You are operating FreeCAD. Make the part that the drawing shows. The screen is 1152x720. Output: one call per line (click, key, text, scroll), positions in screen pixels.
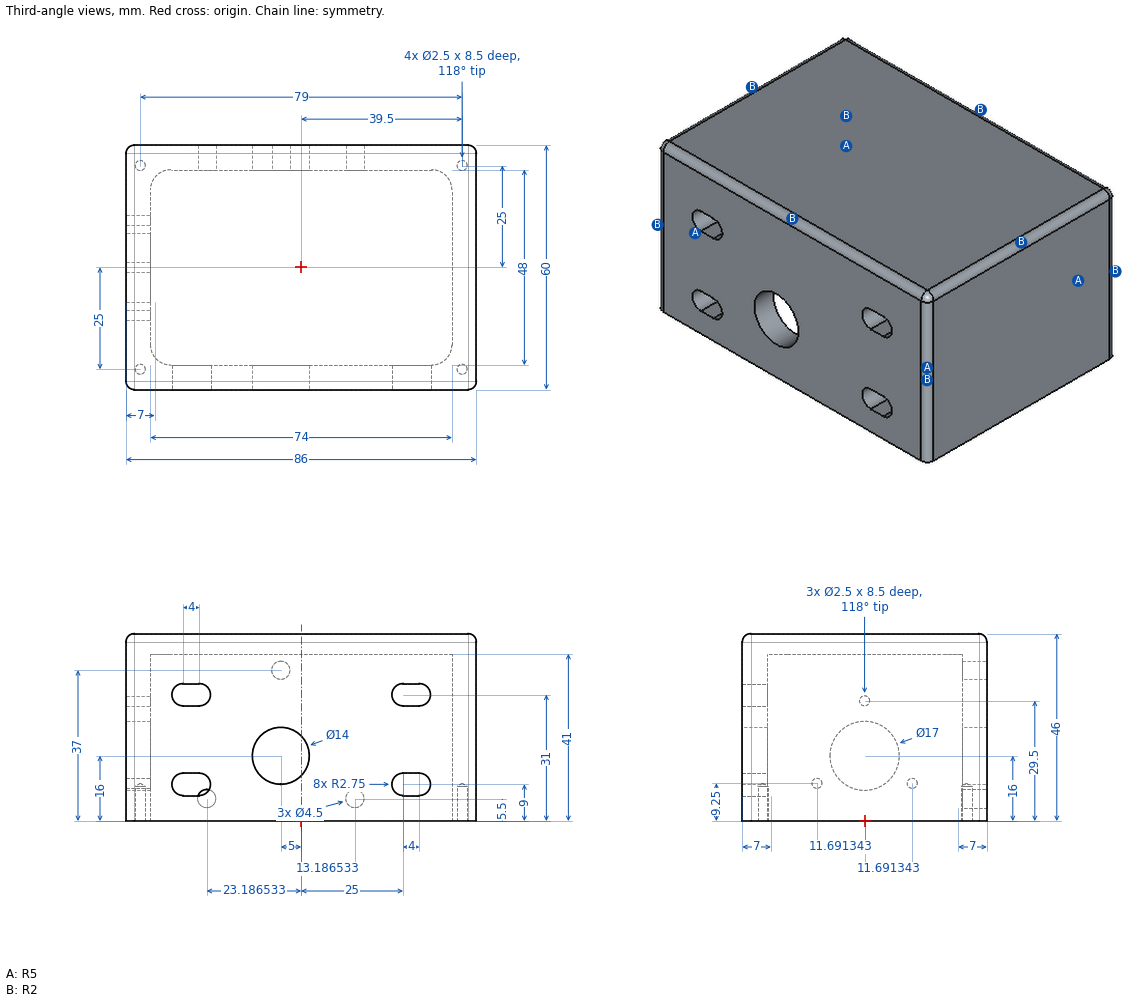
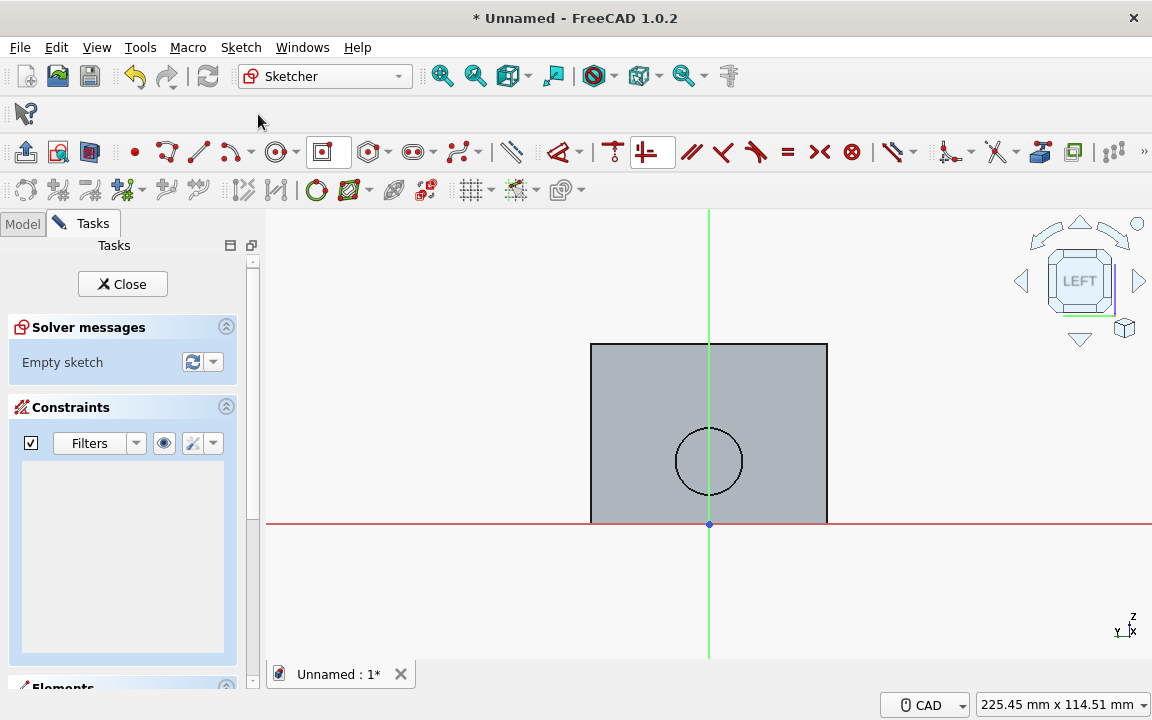
scroll(765, 488, up, 4)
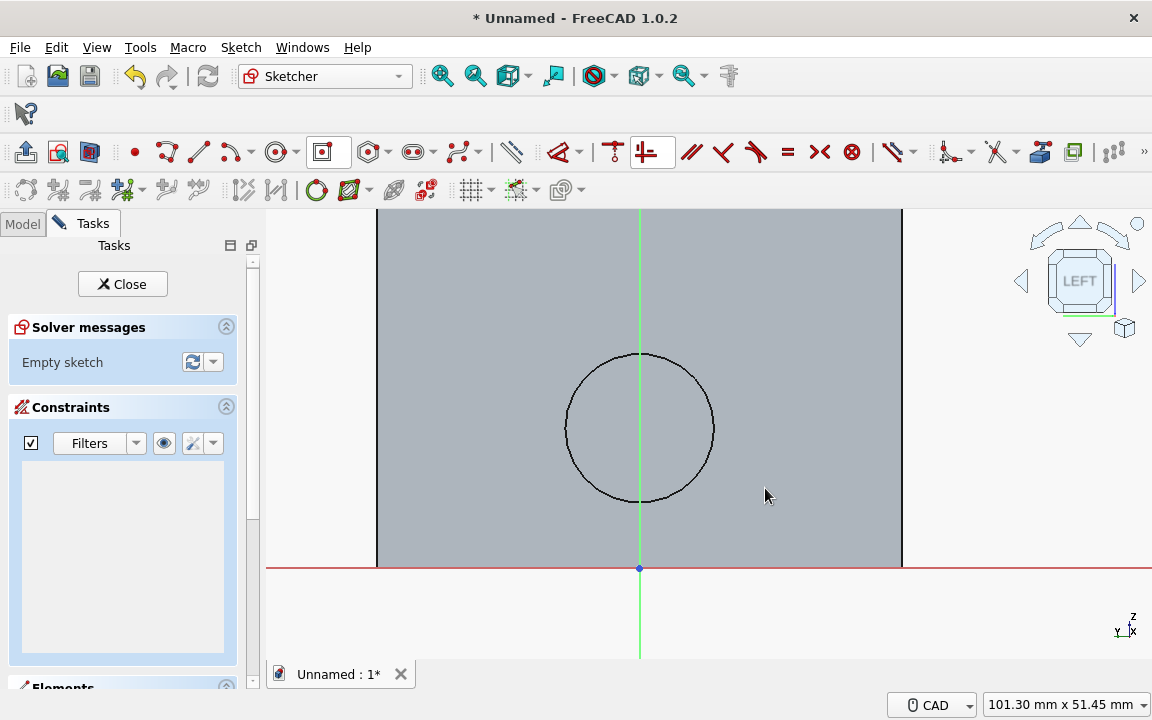
key(g)
key(c)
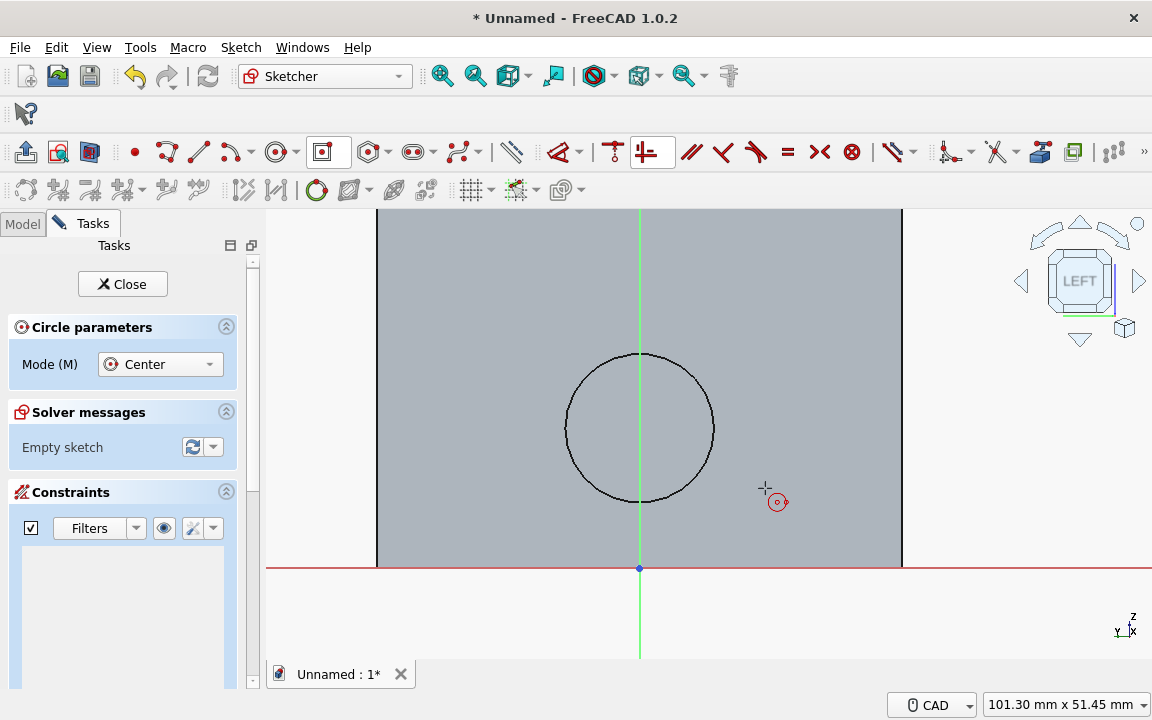
scroll(640, 310, up, 4)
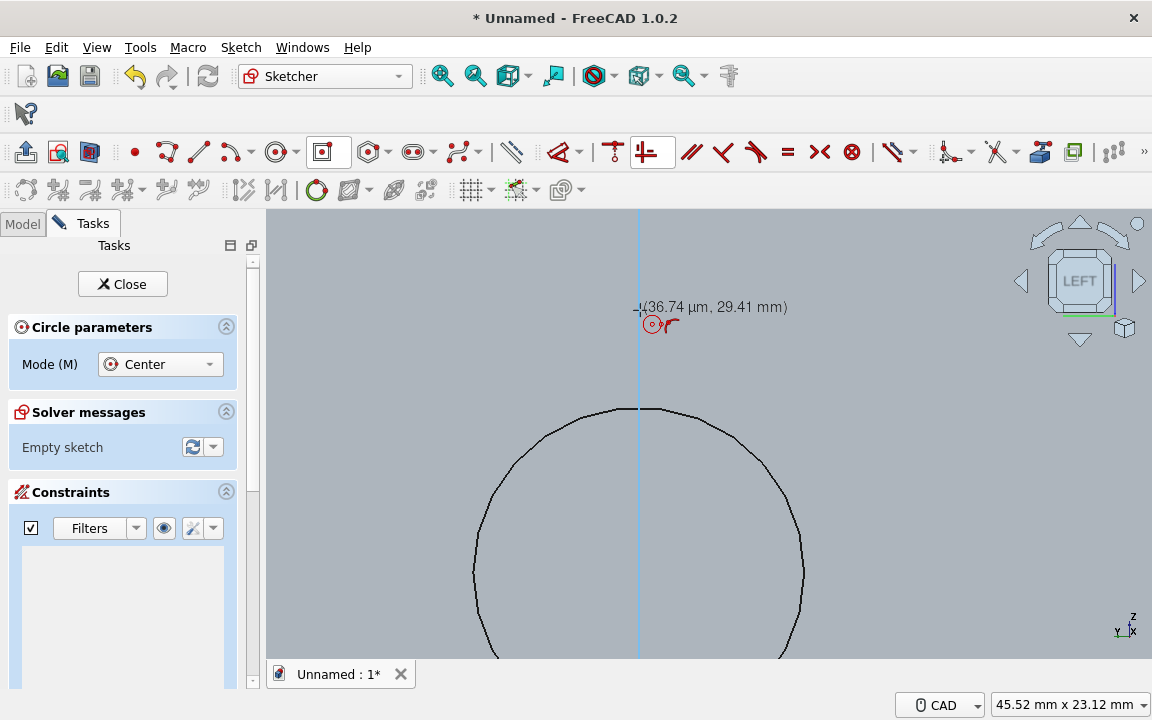
click(639, 310)
click(656, 293)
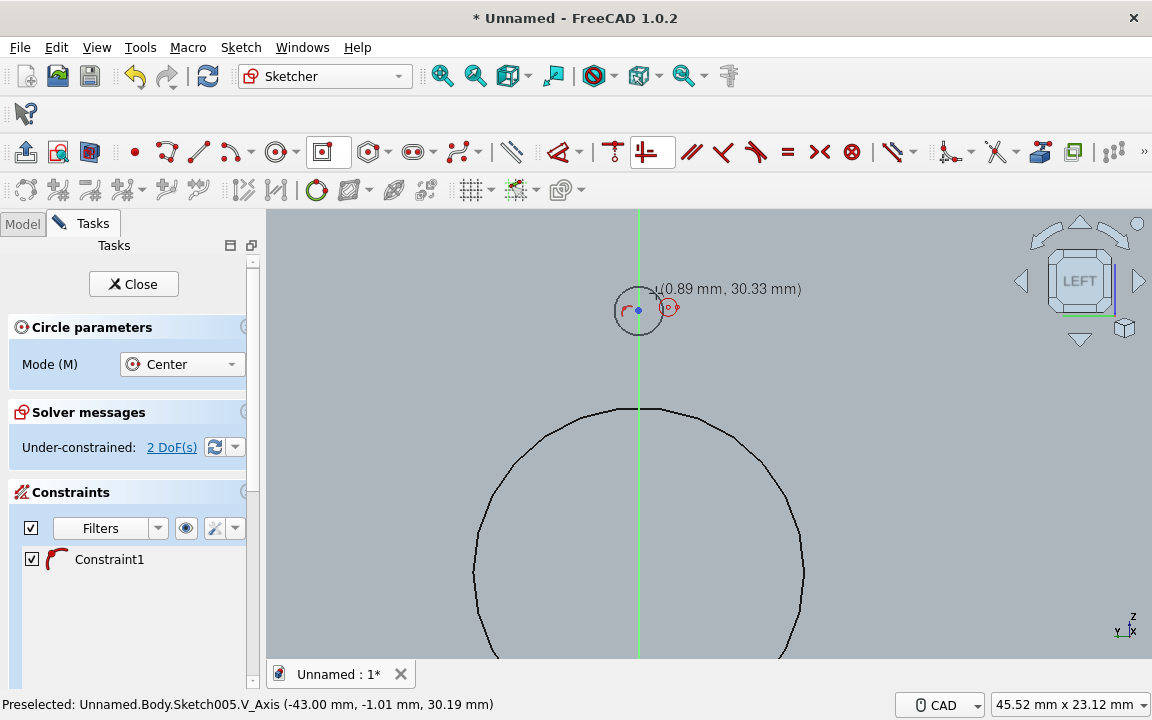
scroll(642, 311, down, 4)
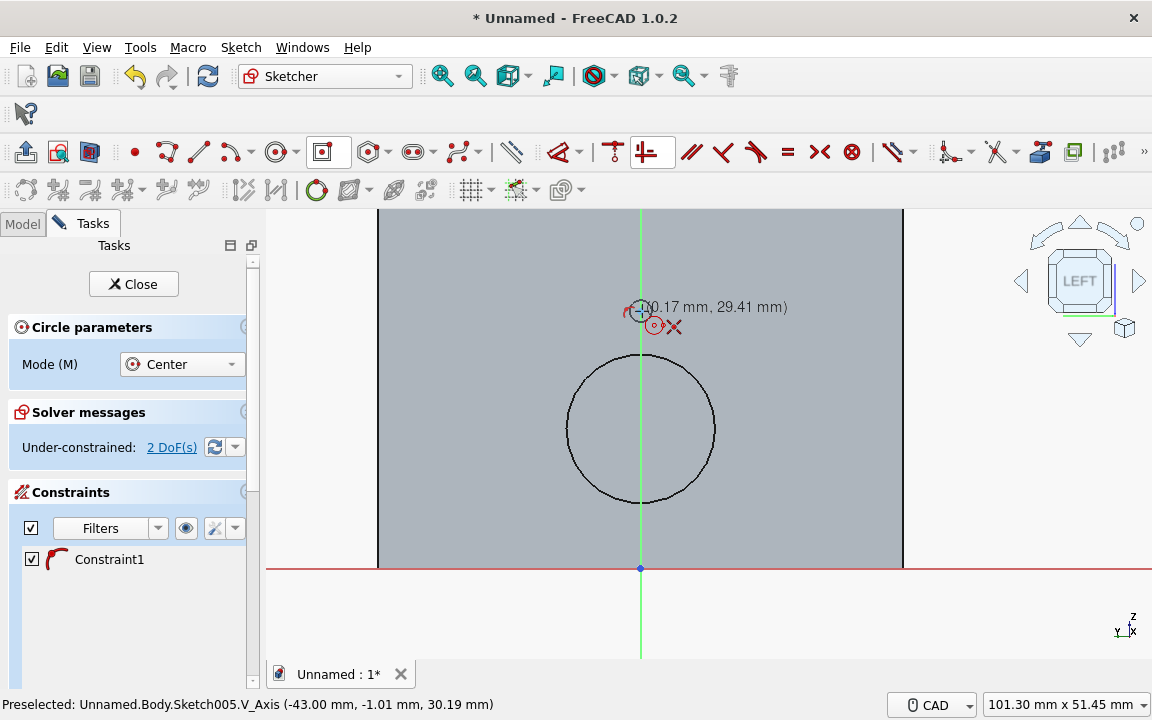
scroll(743, 488, up, 4)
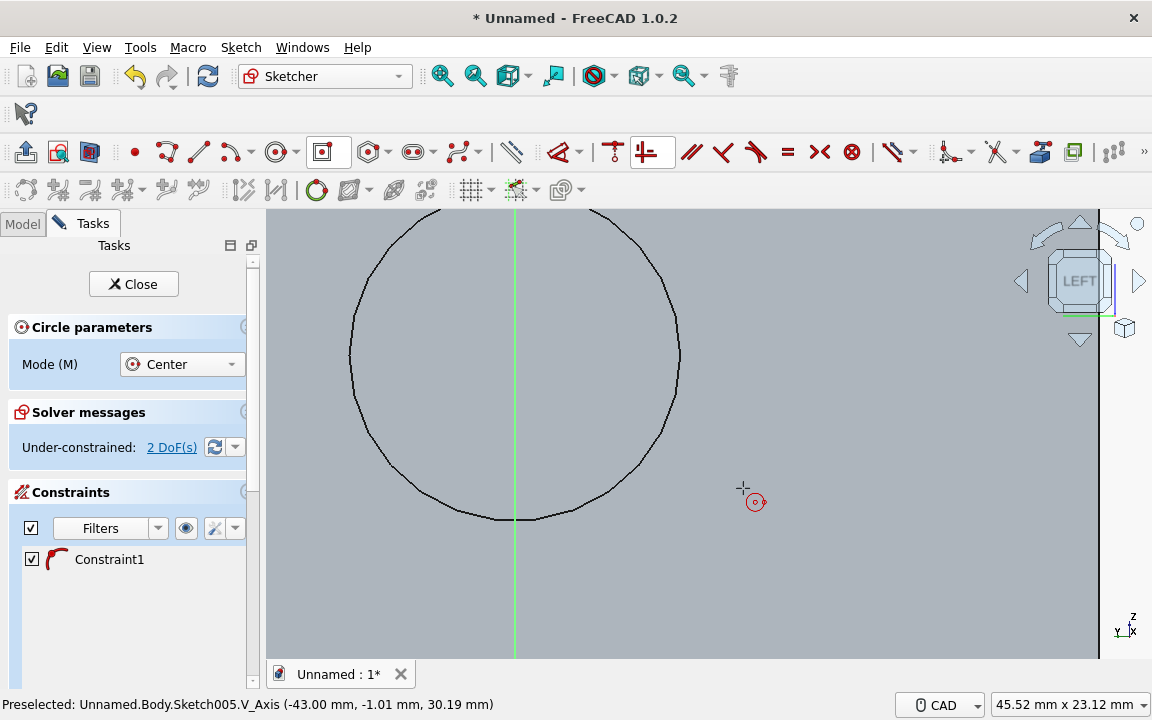
click(742, 487)
click(760, 470)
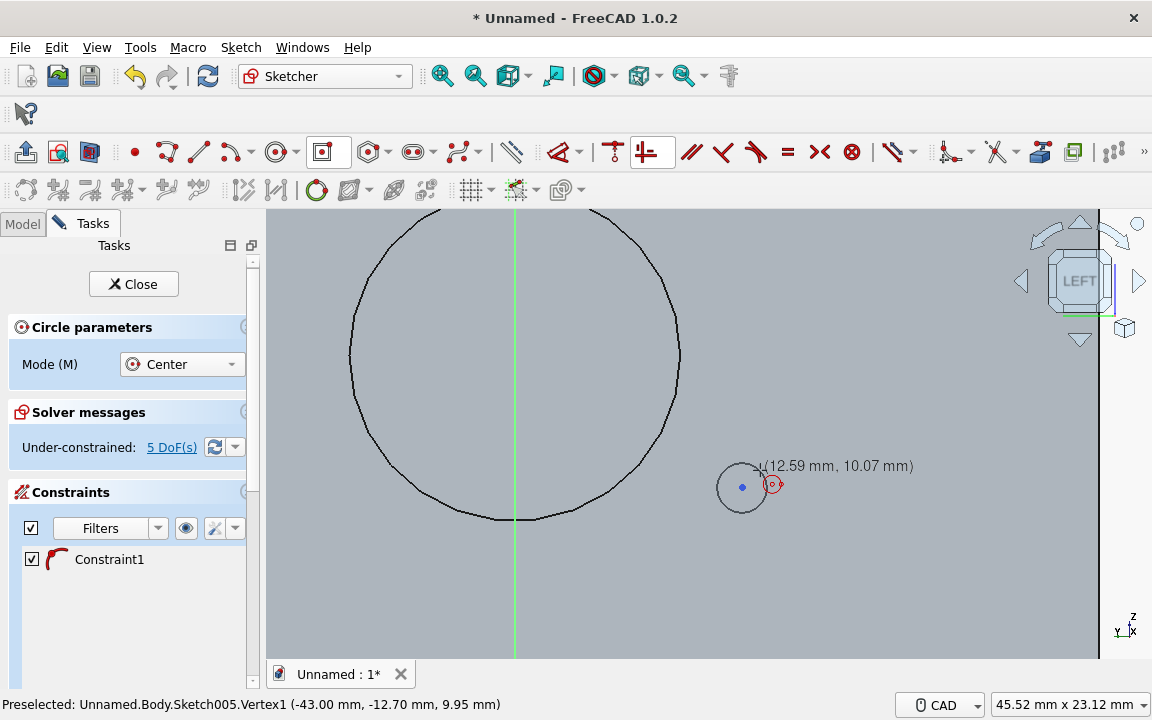
scroll(743, 488, down, 4)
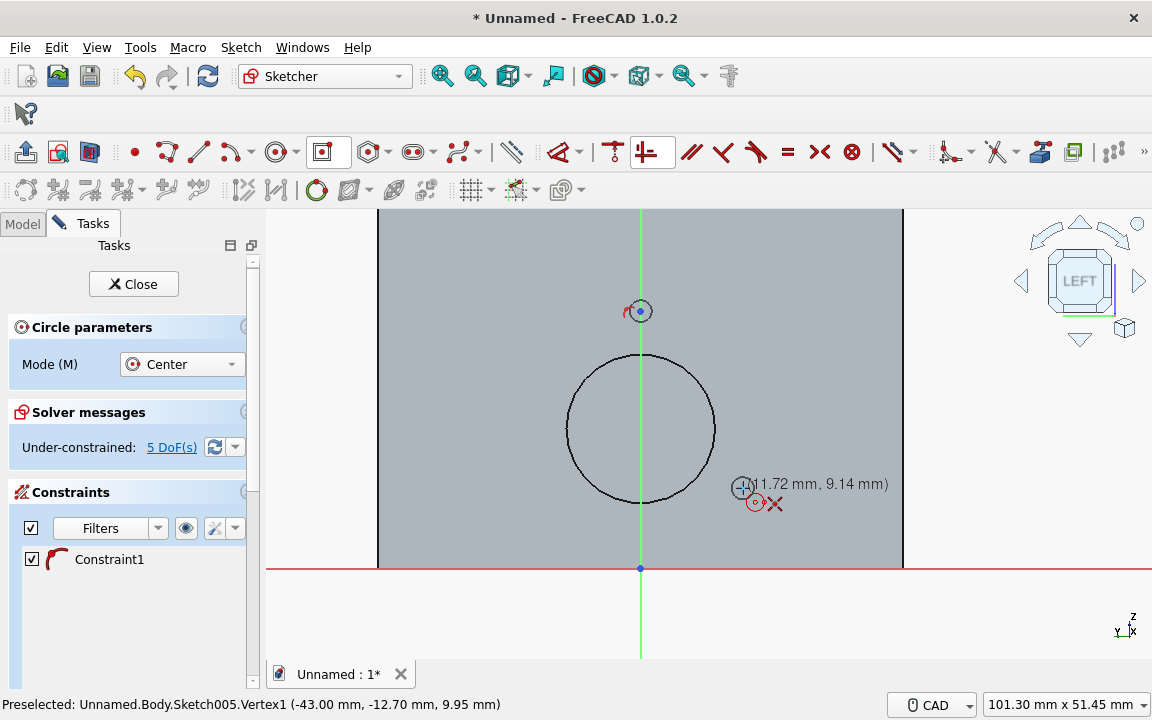
scroll(539, 488, up, 4)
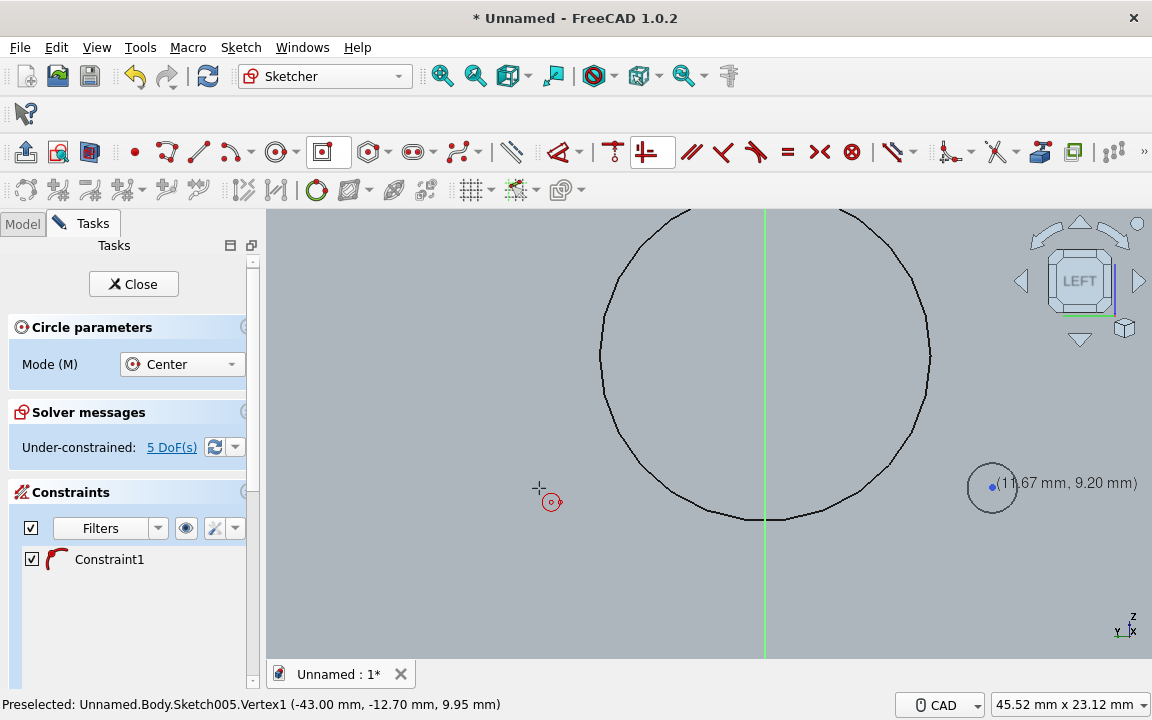
click(538, 487)
click(555, 470)
key(Escape)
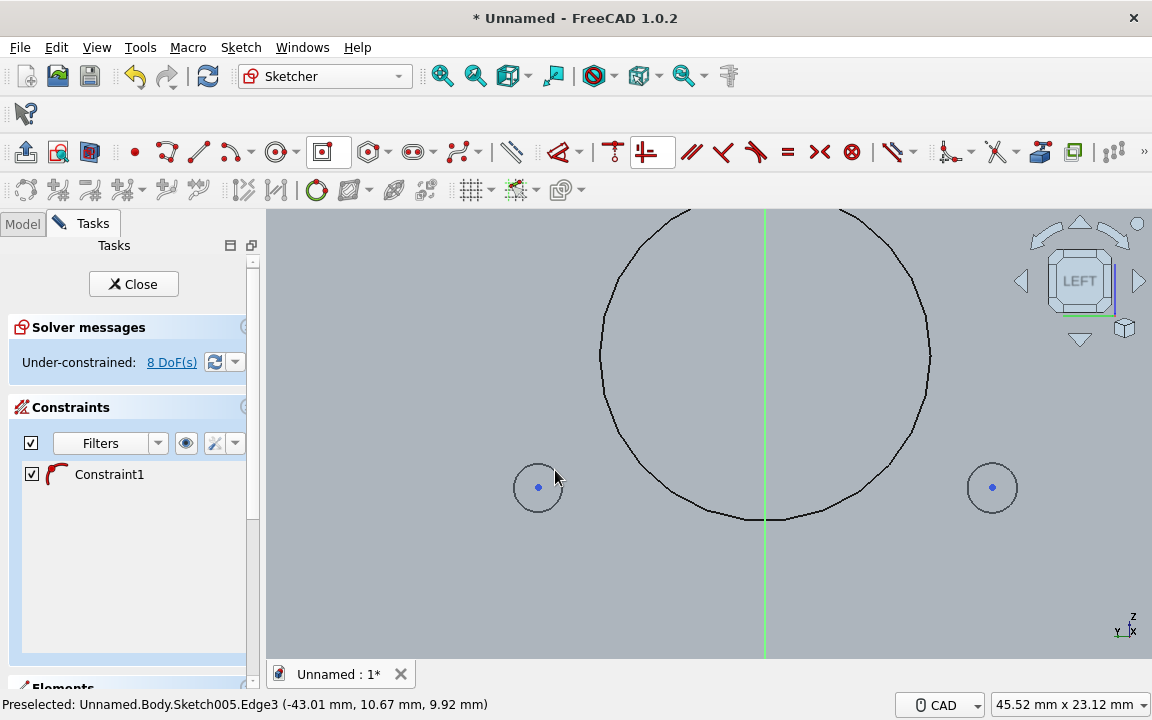
scroll(539, 488, down, 4)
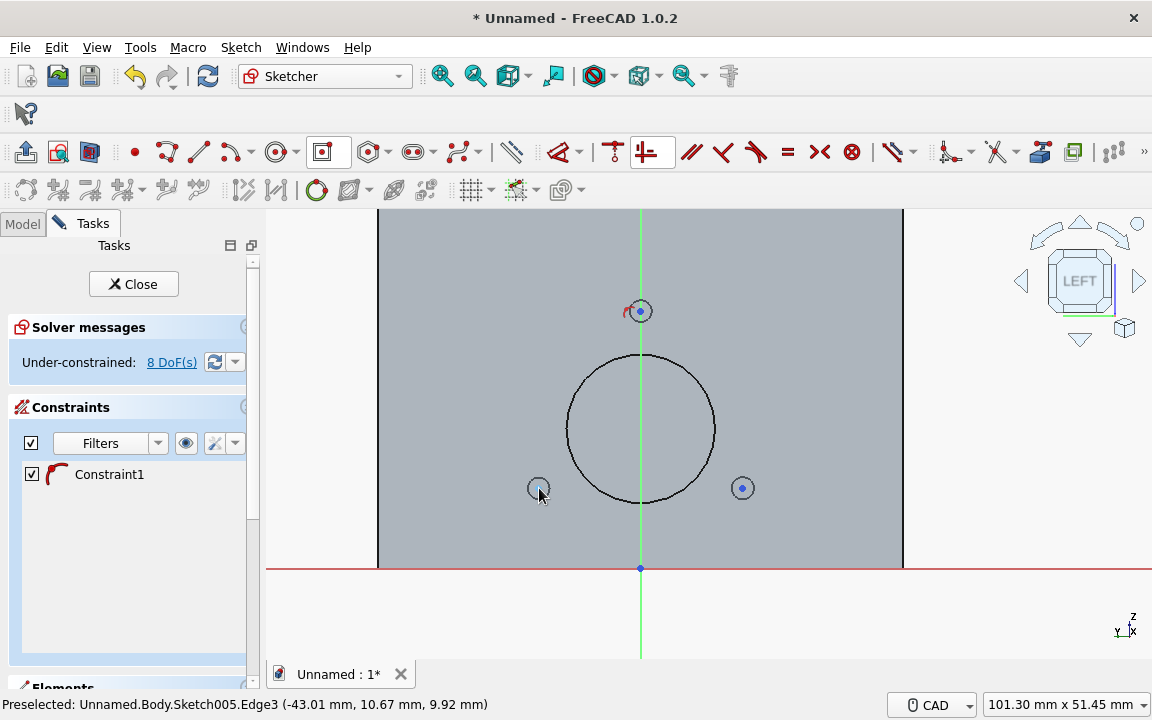
scroll(648, 303, up, 3)